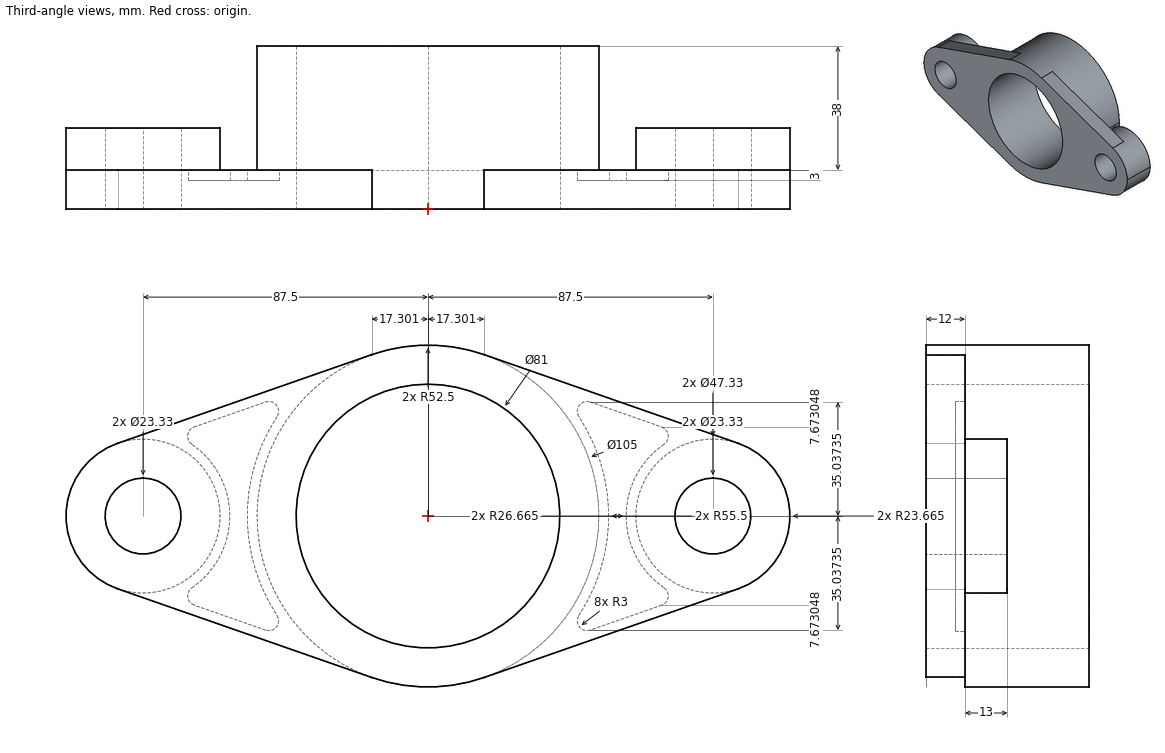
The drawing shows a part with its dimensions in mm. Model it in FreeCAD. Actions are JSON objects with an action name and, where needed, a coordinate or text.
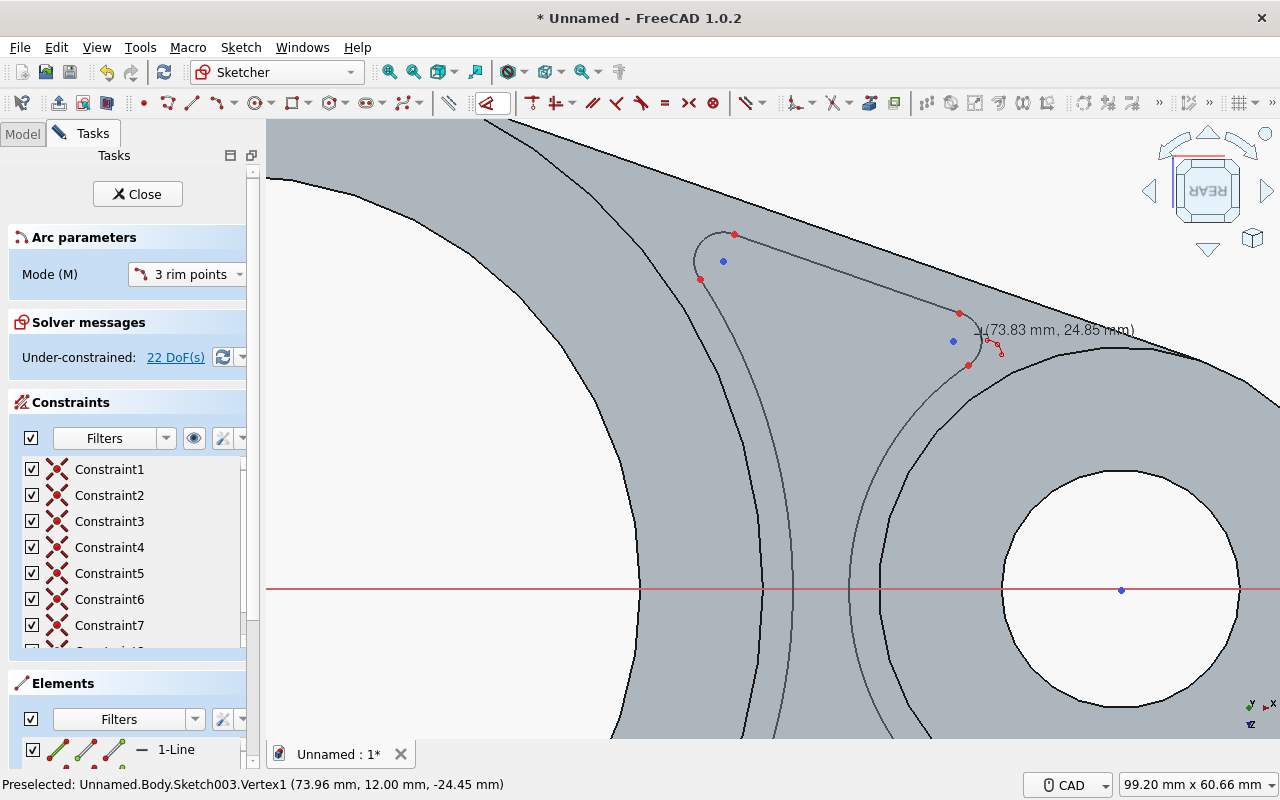
{"action": "left_click", "coordinate": [192, 104]}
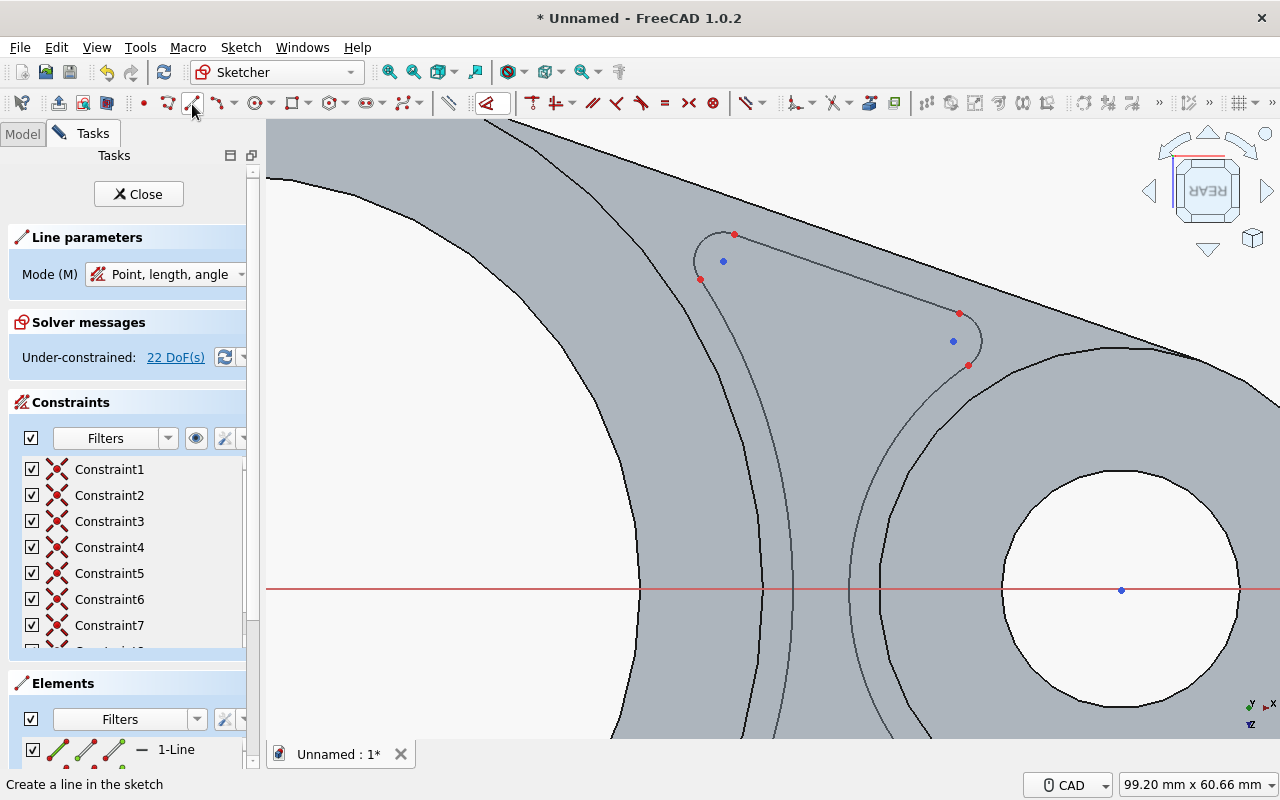
{"action": "scroll", "coordinate": [983, 336], "scroll_direction": "down", "scroll_amount": 5}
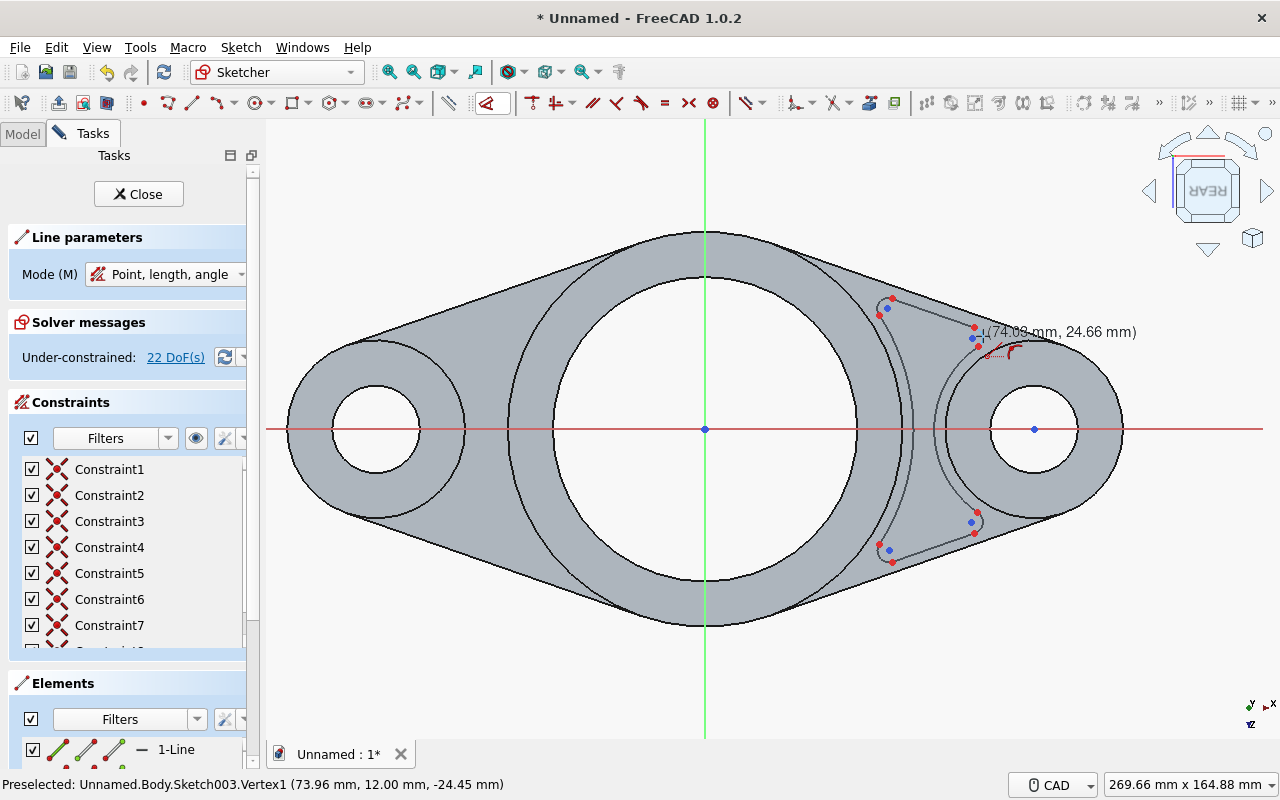
{"action": "left_click", "coordinate": [435, 532]}
{"action": "left_click", "coordinate": [518, 561]}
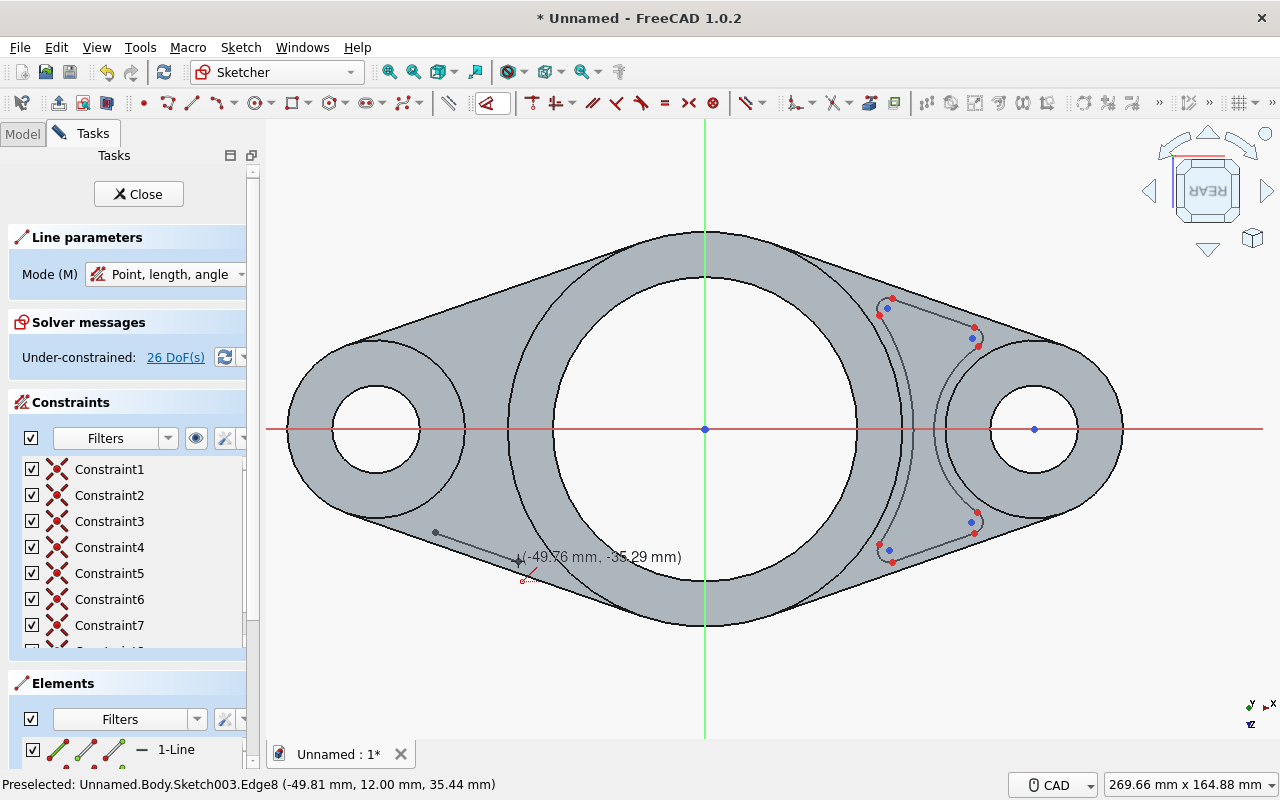
{"action": "left_click", "coordinate": [518, 298]}
{"action": "left_click", "coordinate": [435, 326]}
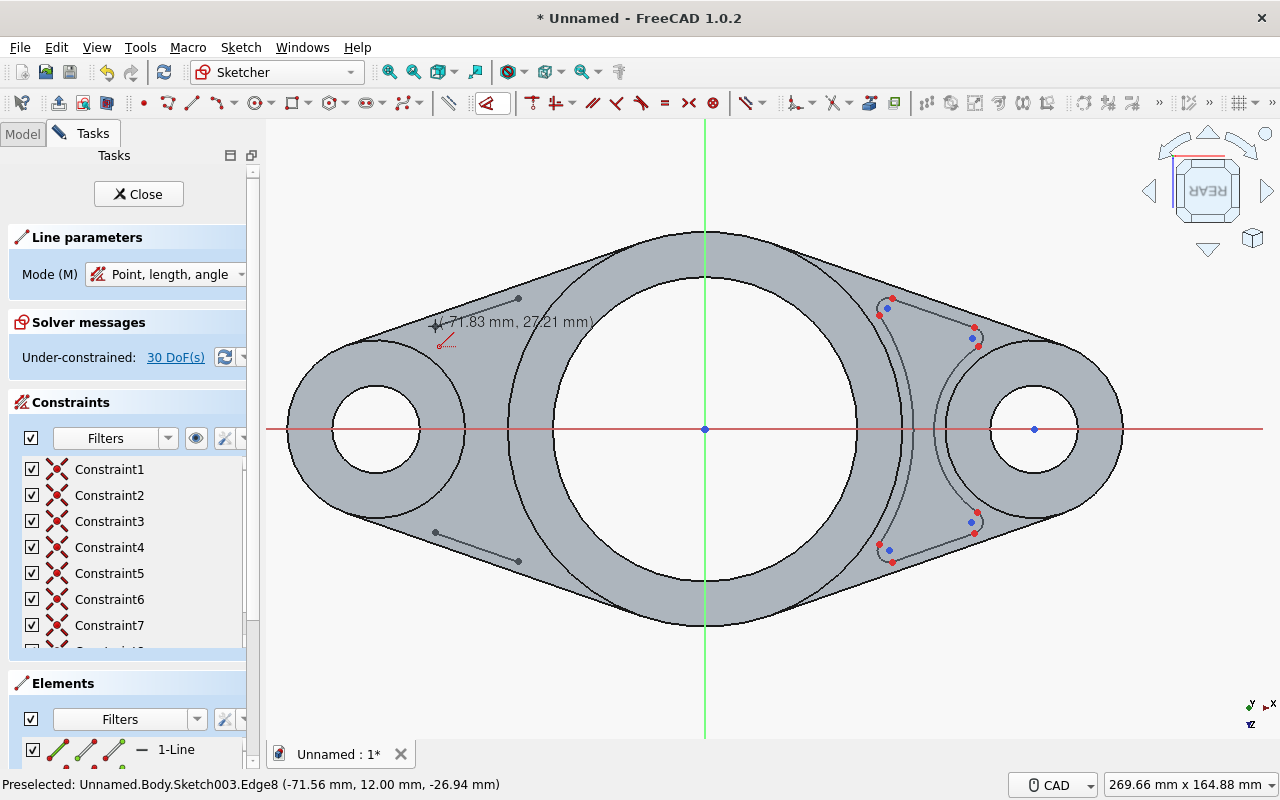
{"action": "left_click", "coordinate": [218, 104]}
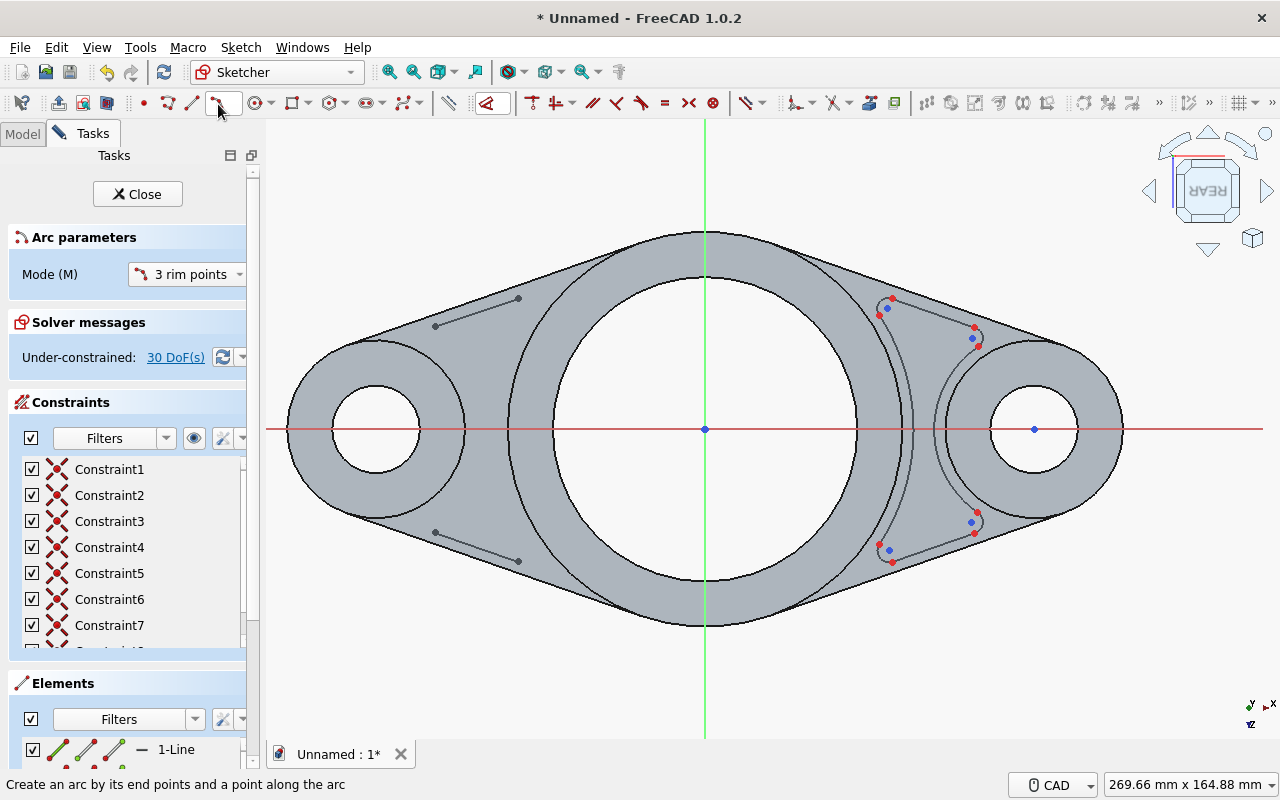
{"action": "left_click", "coordinate": [518, 562]}
{"action": "left_click", "coordinate": [531, 544]}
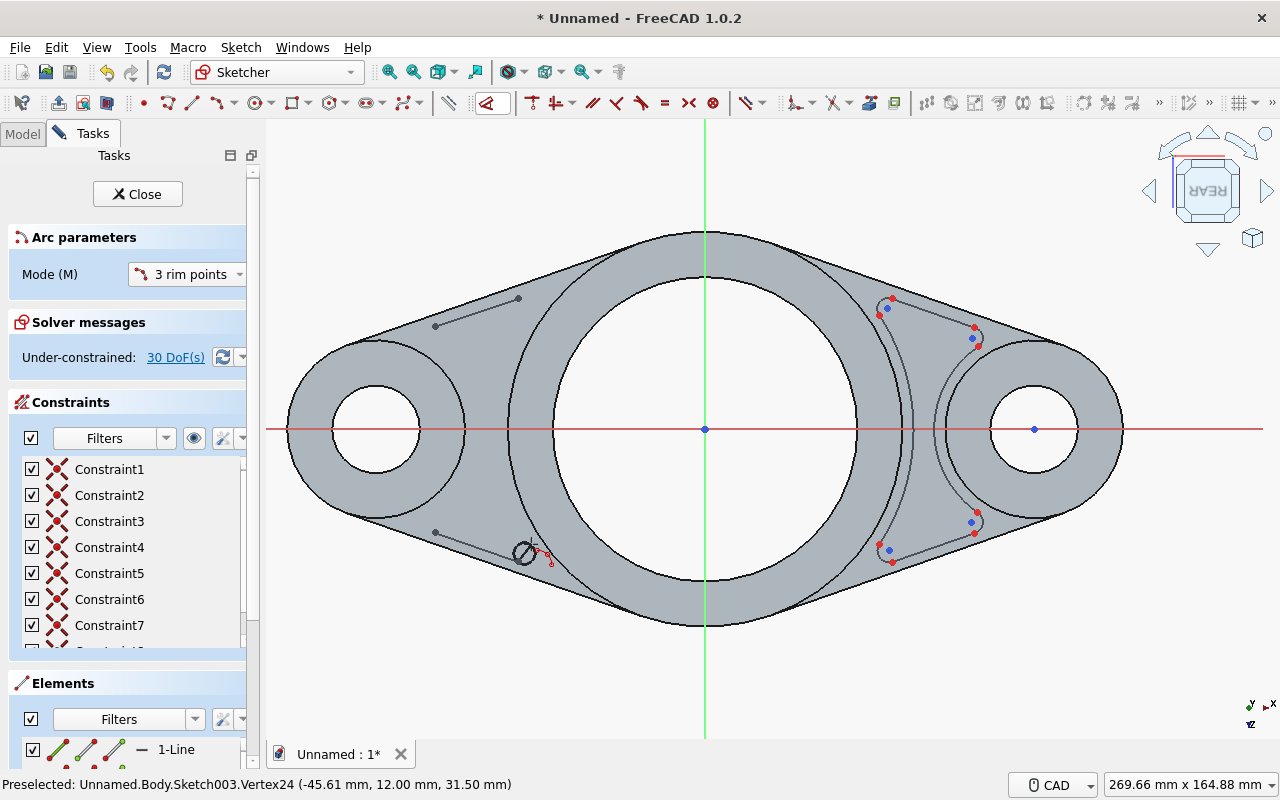
{"action": "scroll", "coordinate": [530, 557], "scroll_direction": "up", "scroll_amount": 4}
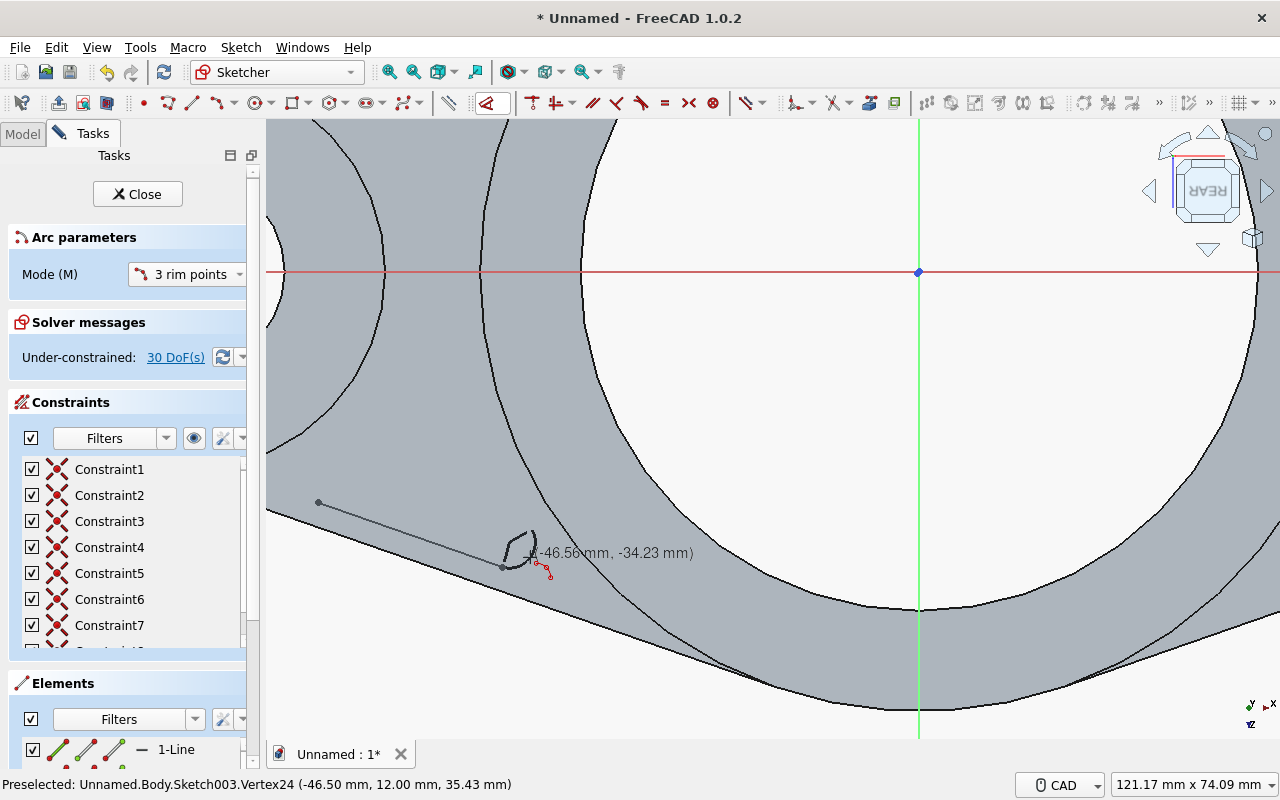
{"action": "left_click", "coordinate": [530, 557]}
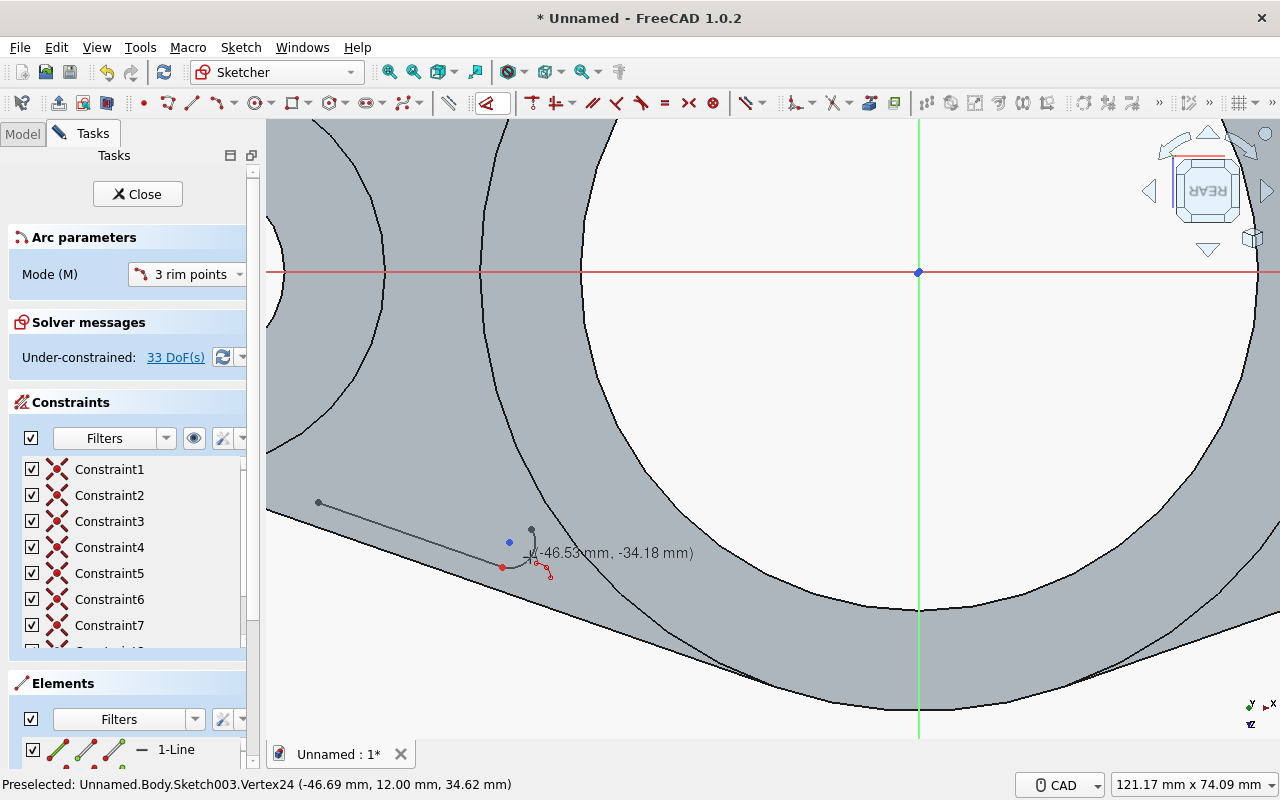
{"action": "left_click", "coordinate": [532, 529]}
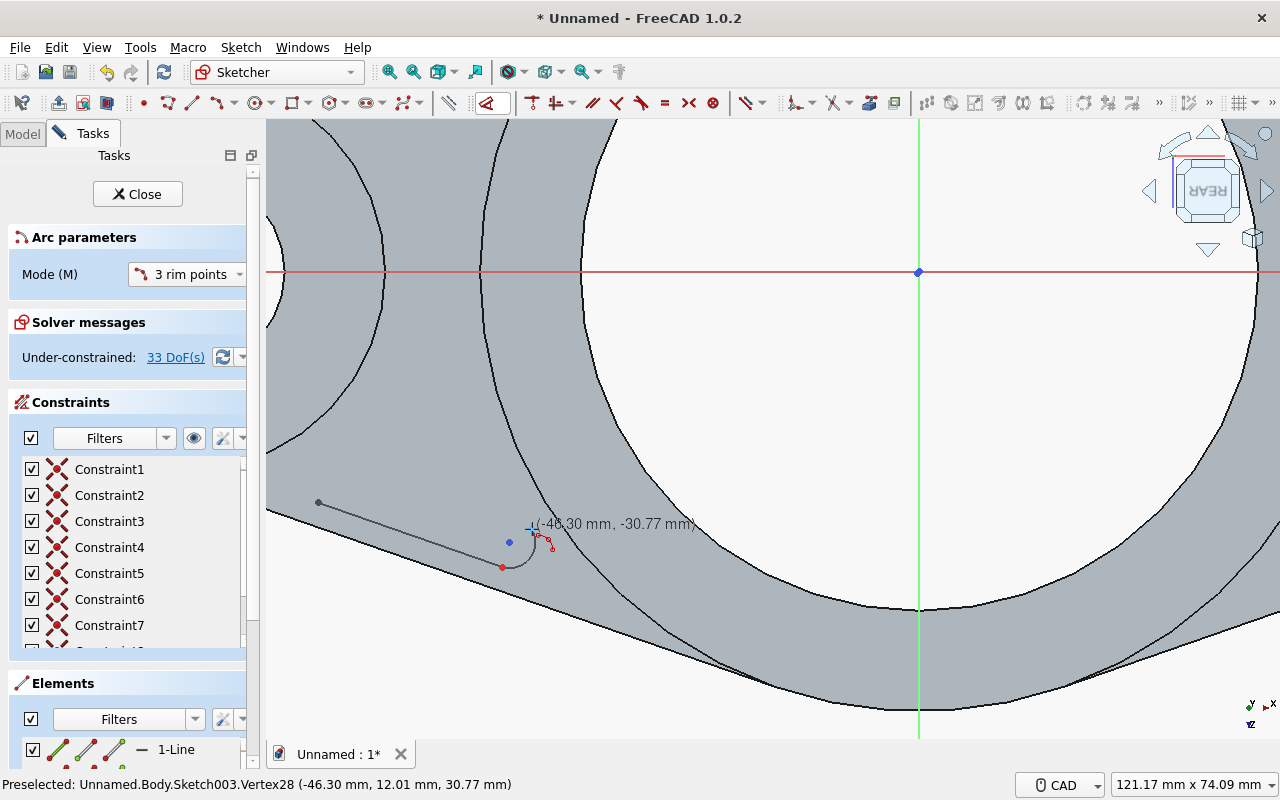
{"action": "scroll", "coordinate": [529, 557], "scroll_direction": "down", "scroll_amount": 4}